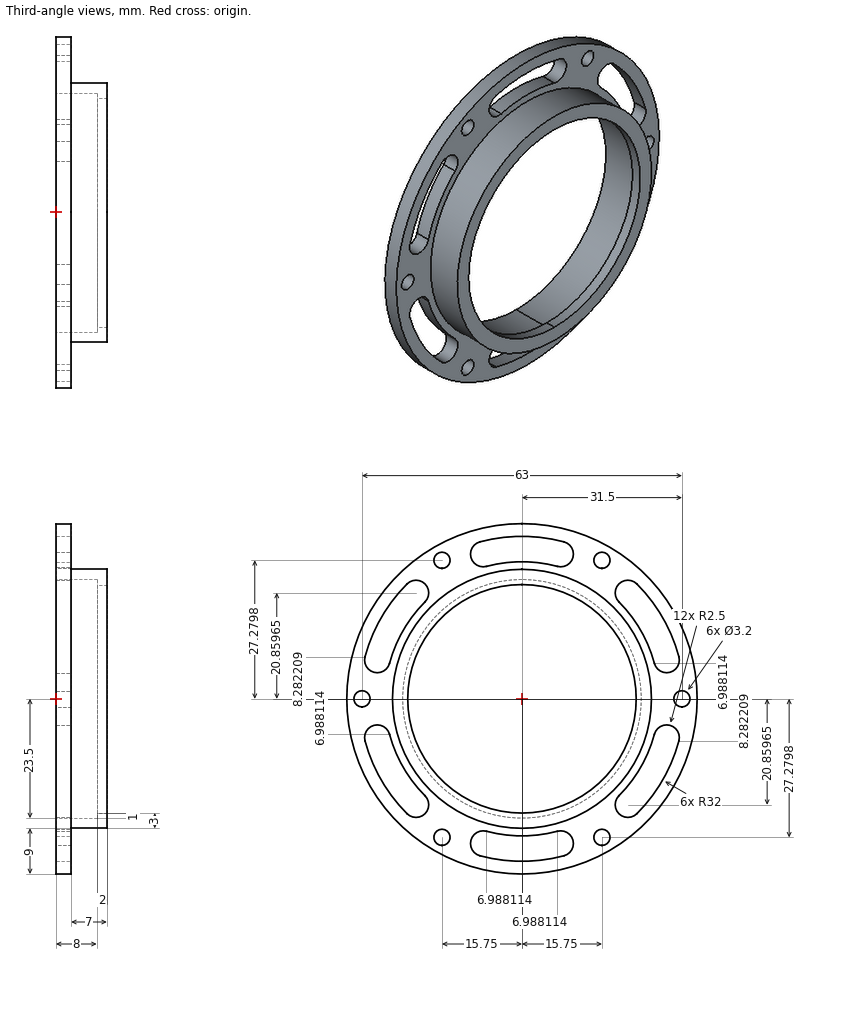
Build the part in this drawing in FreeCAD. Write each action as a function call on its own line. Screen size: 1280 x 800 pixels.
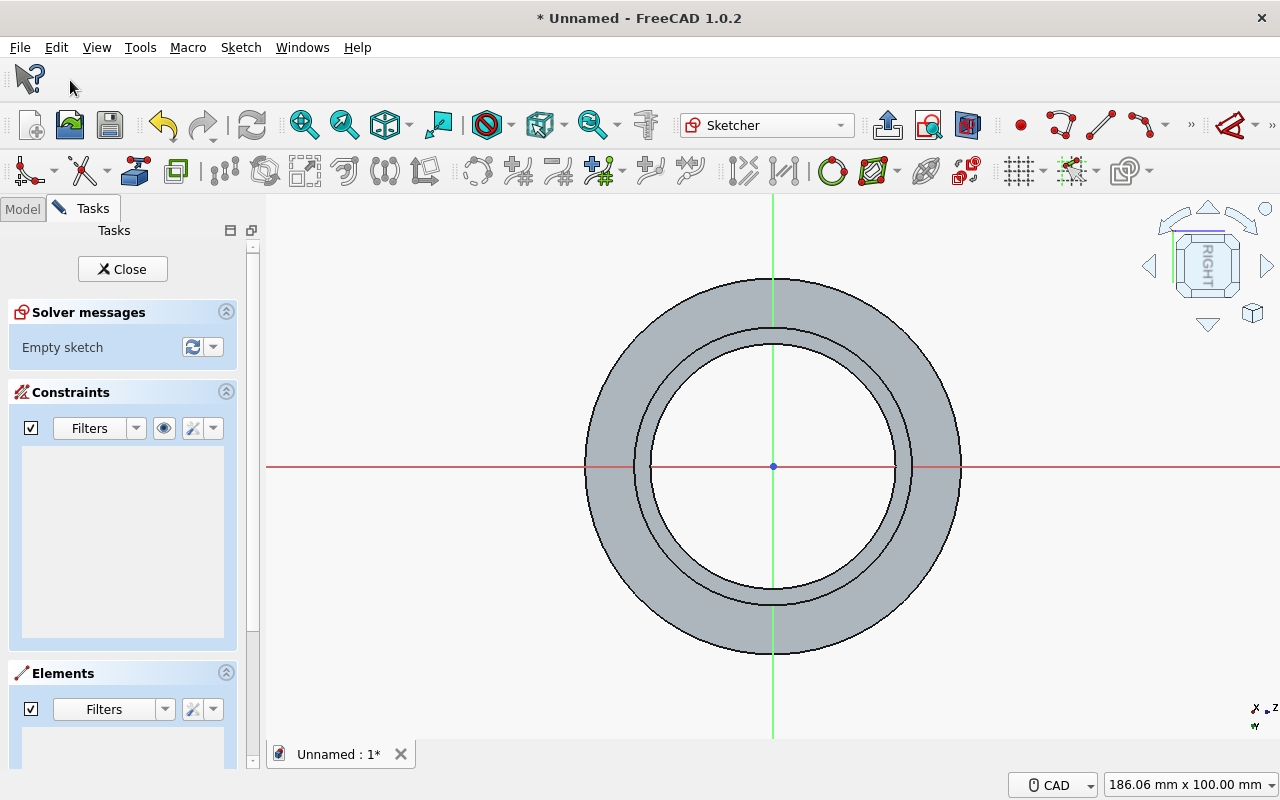
key(q)
key(s)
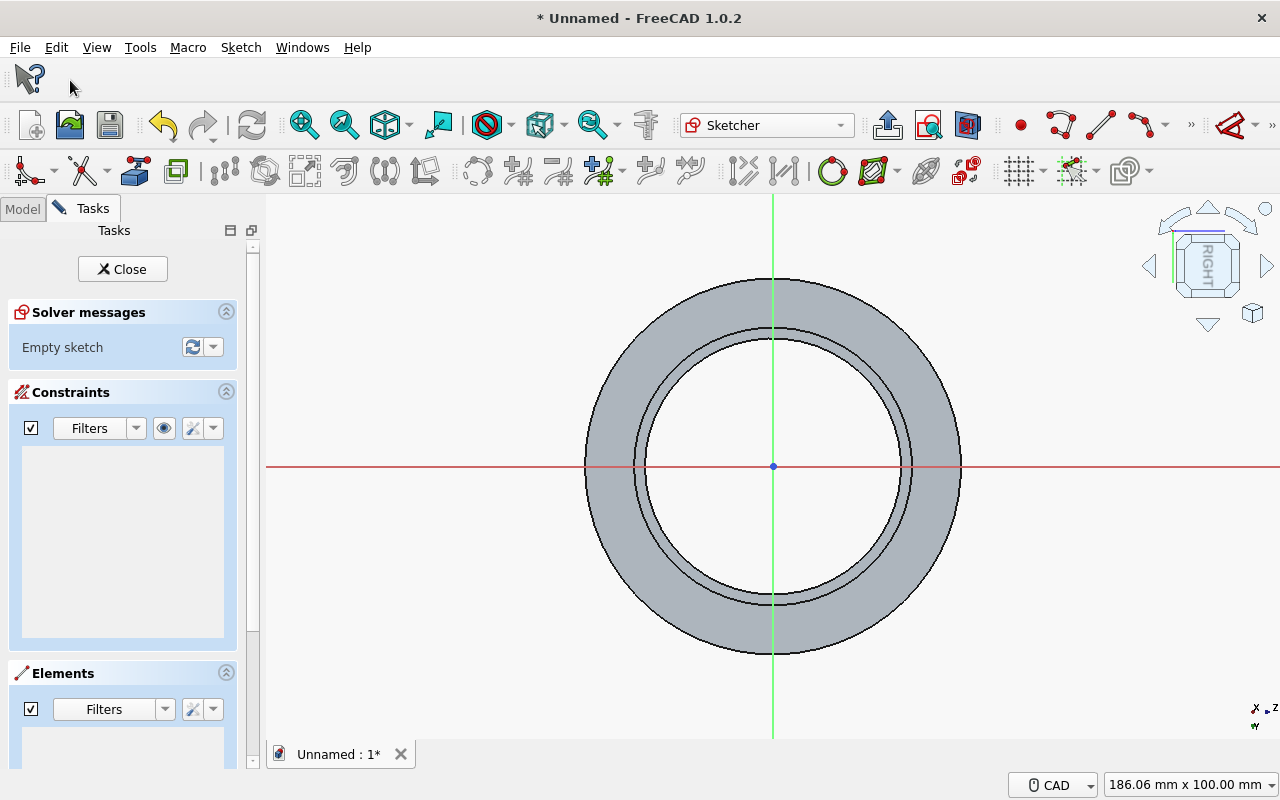
key(g)
key(c)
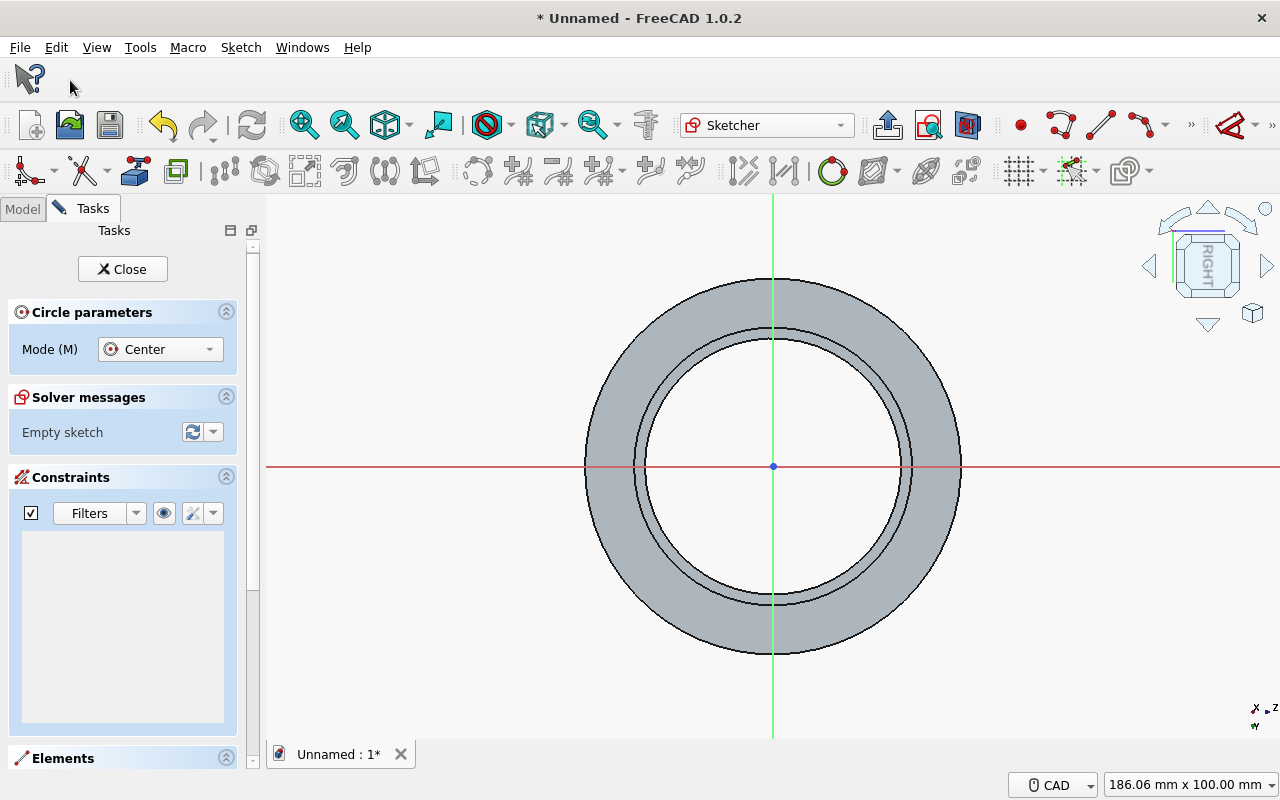
scroll(773, 638, up, 5)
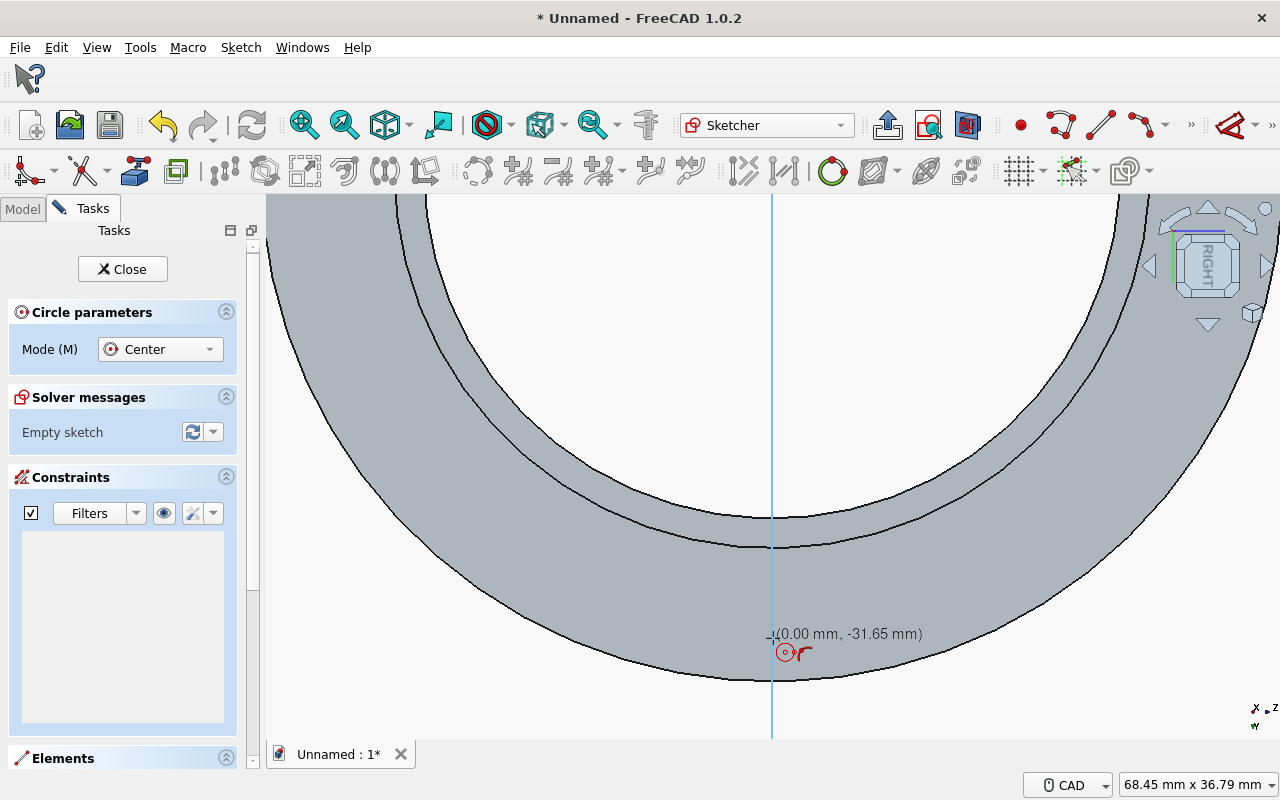
click(772, 637)
click(789, 620)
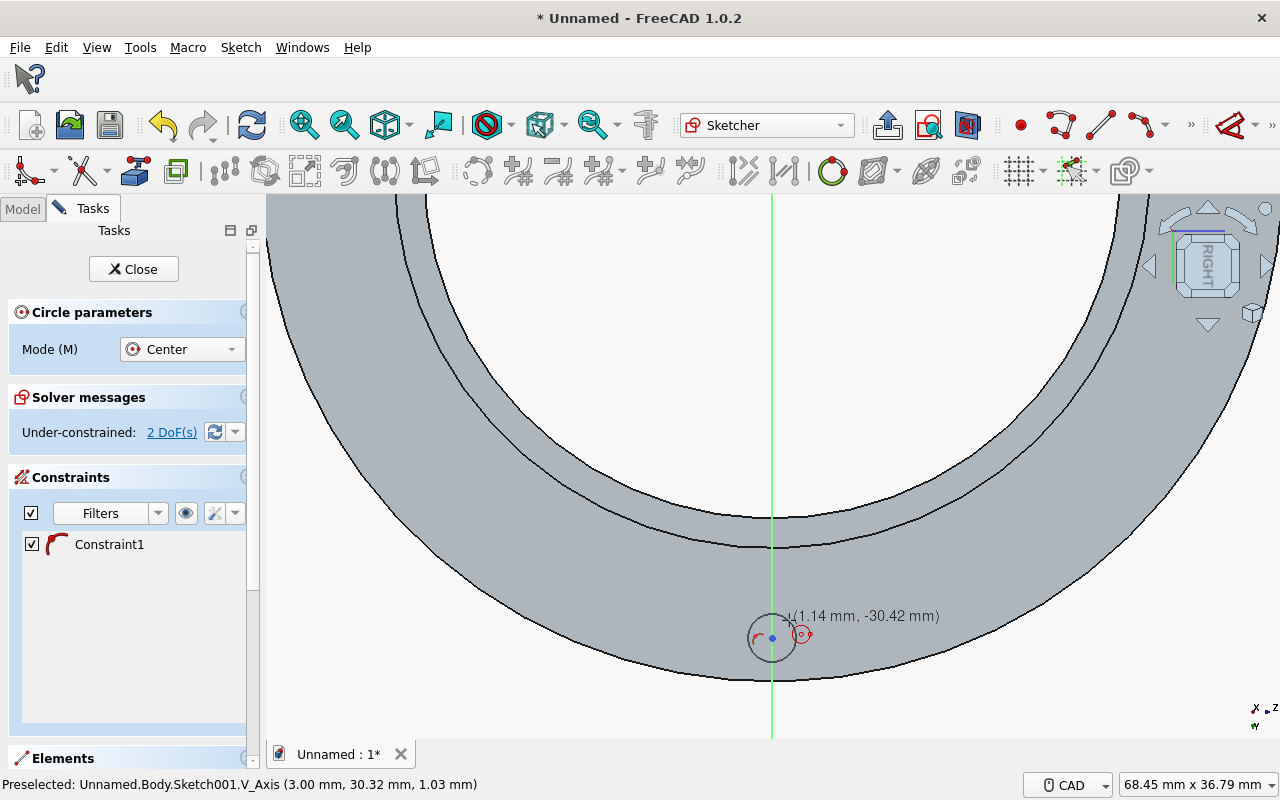
click(368, 404)
click(385, 387)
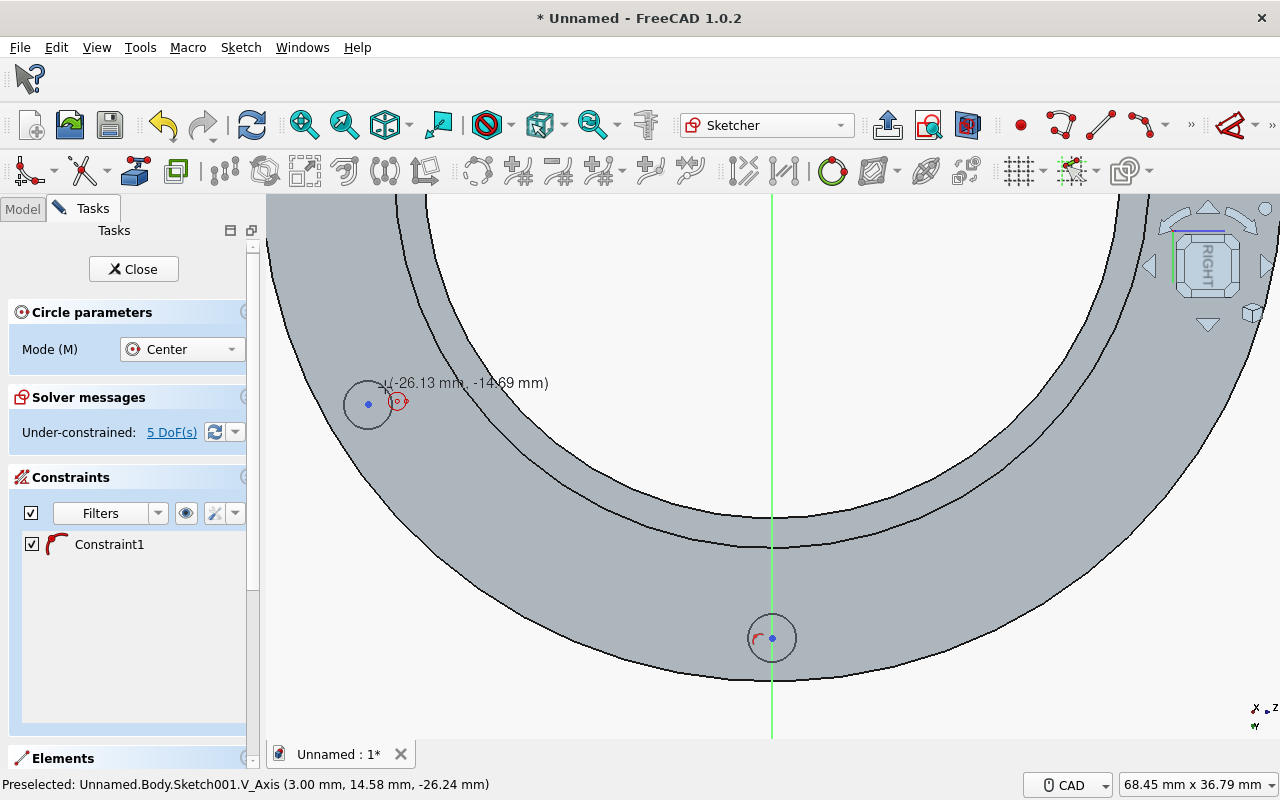
scroll(665, 639, down, 5)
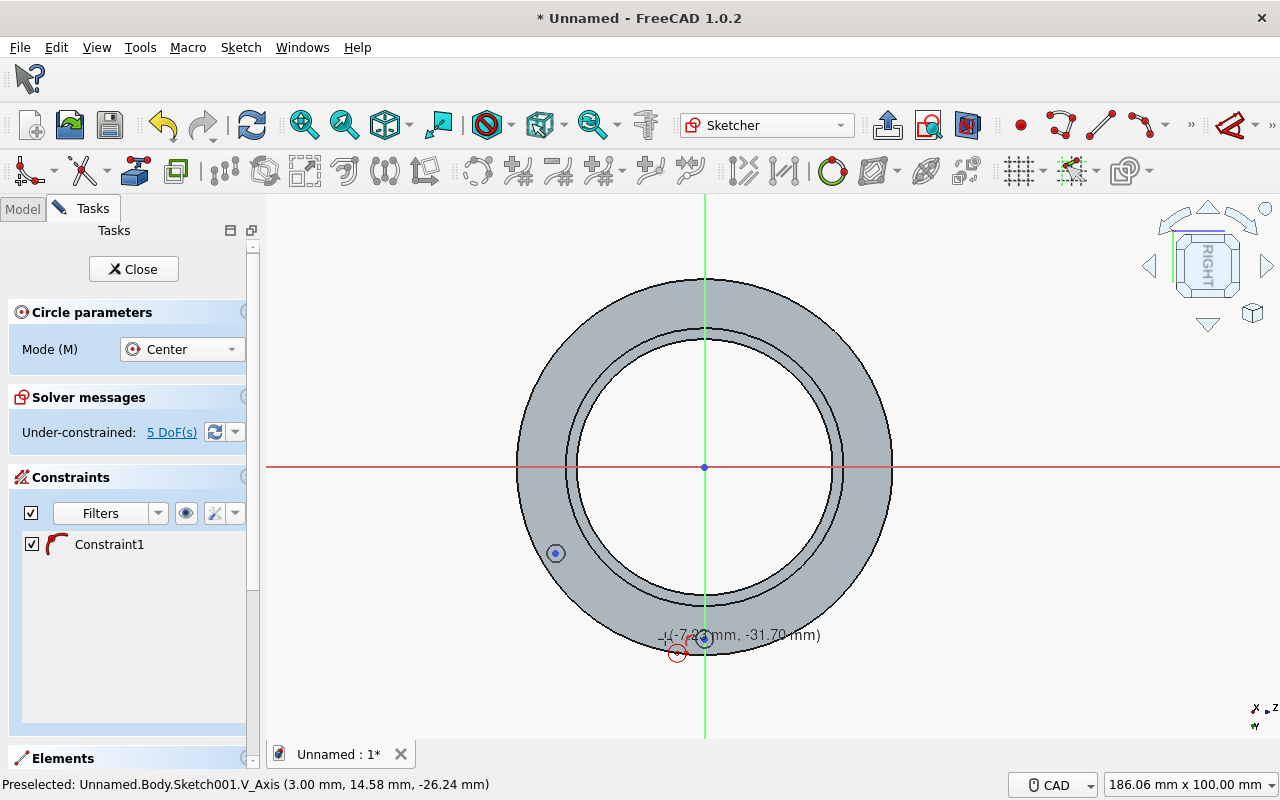
scroll(556, 381, up, 5)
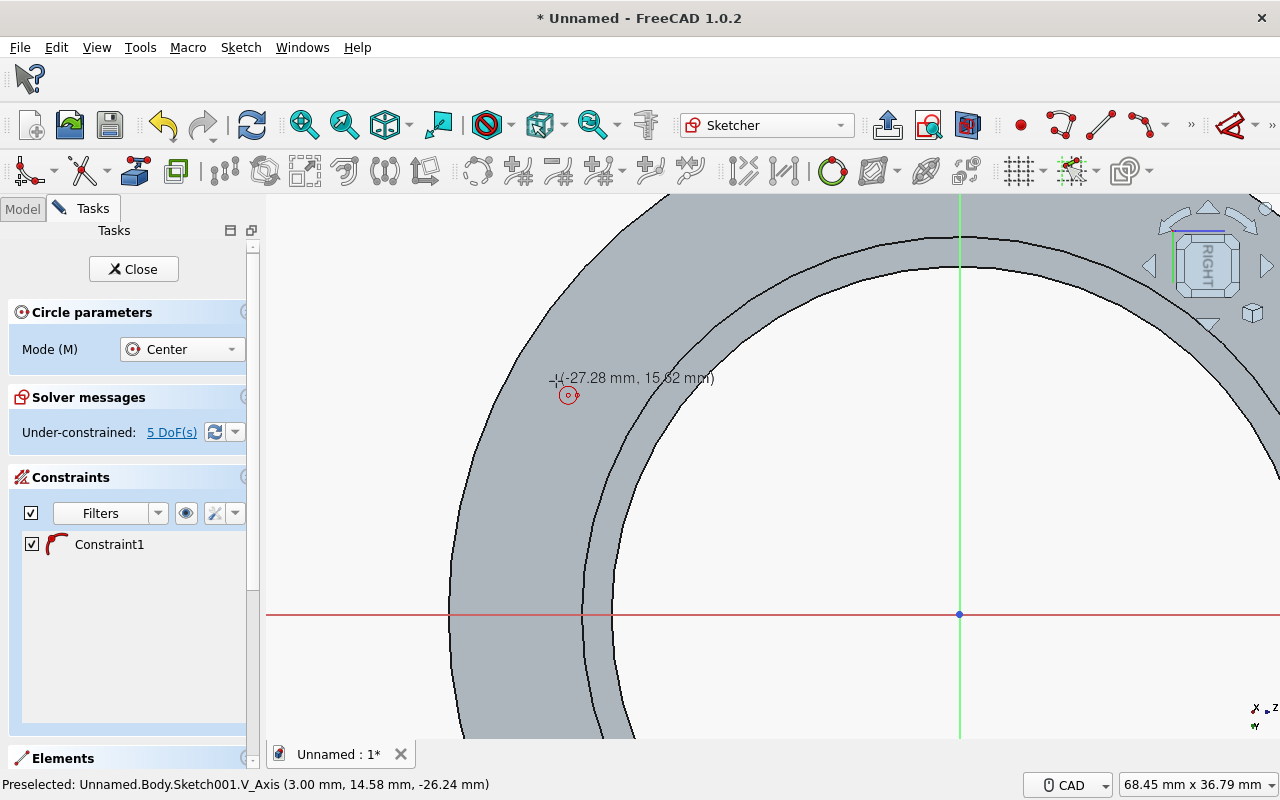
click(555, 381)
click(572, 364)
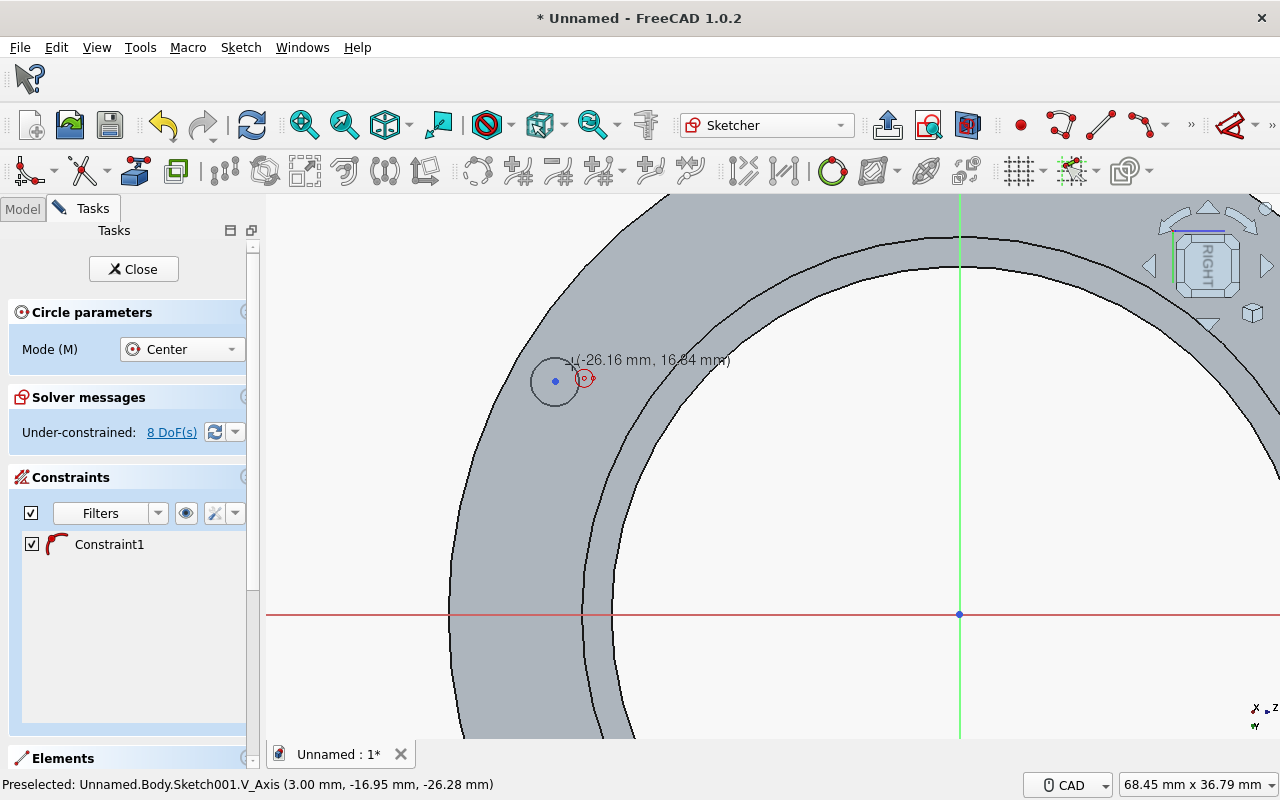
scroll(556, 380, down, 5)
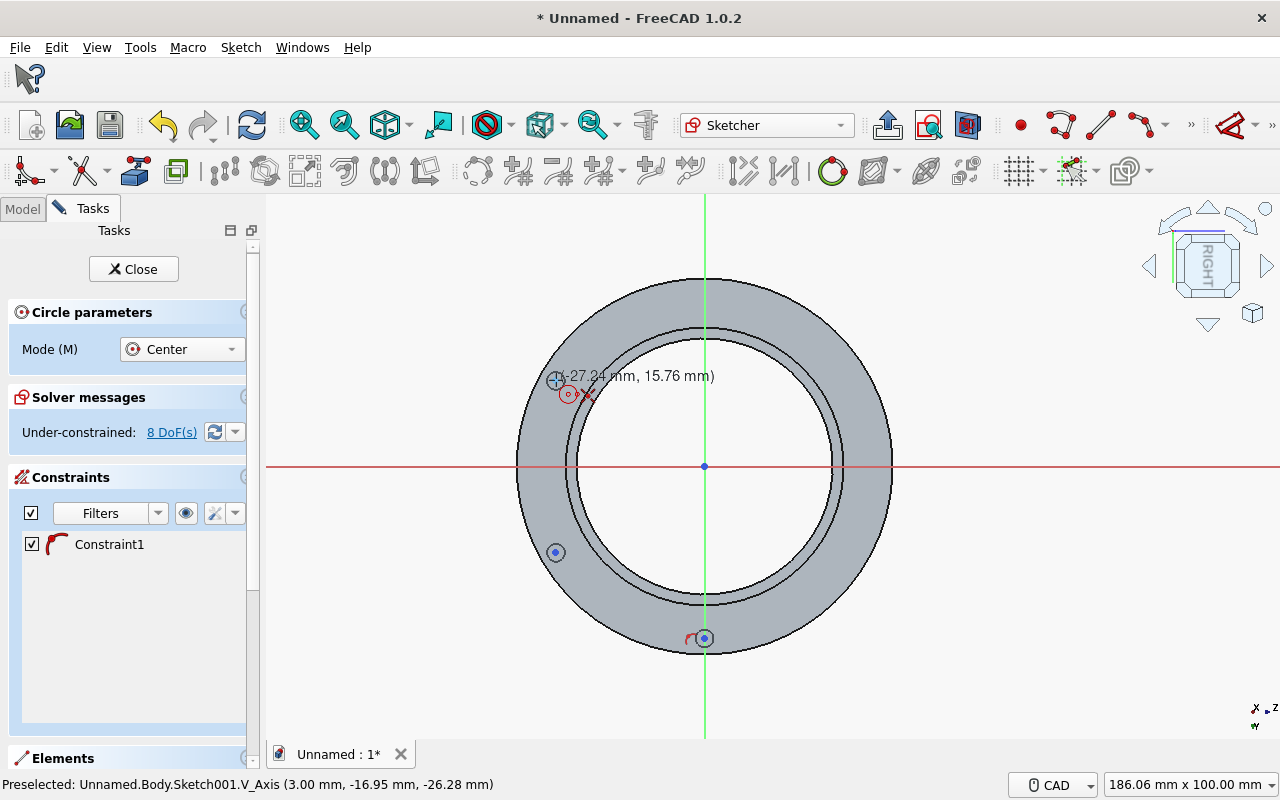
scroll(705, 295, up, 5)